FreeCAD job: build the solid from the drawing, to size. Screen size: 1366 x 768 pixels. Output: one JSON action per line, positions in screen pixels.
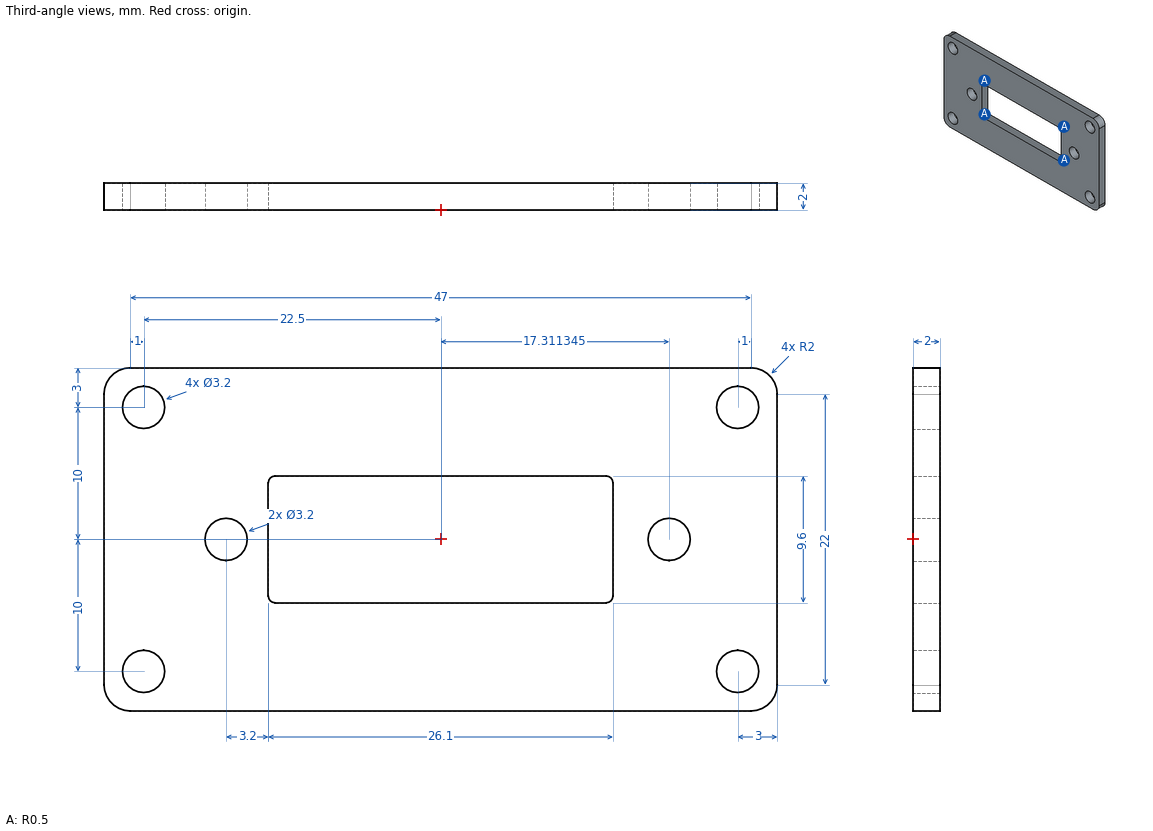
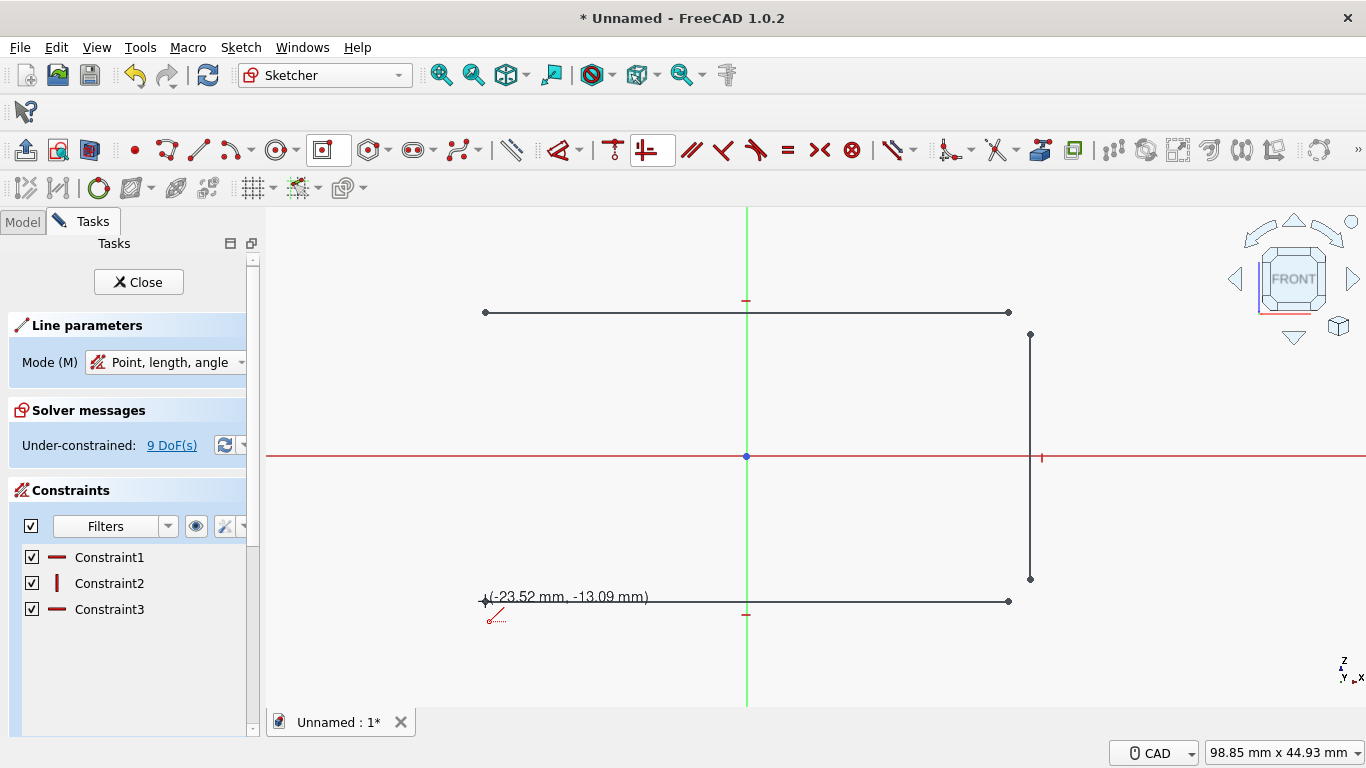
{"action": "left_click", "coordinate": [463, 579]}
{"action": "left_click", "coordinate": [463, 334]}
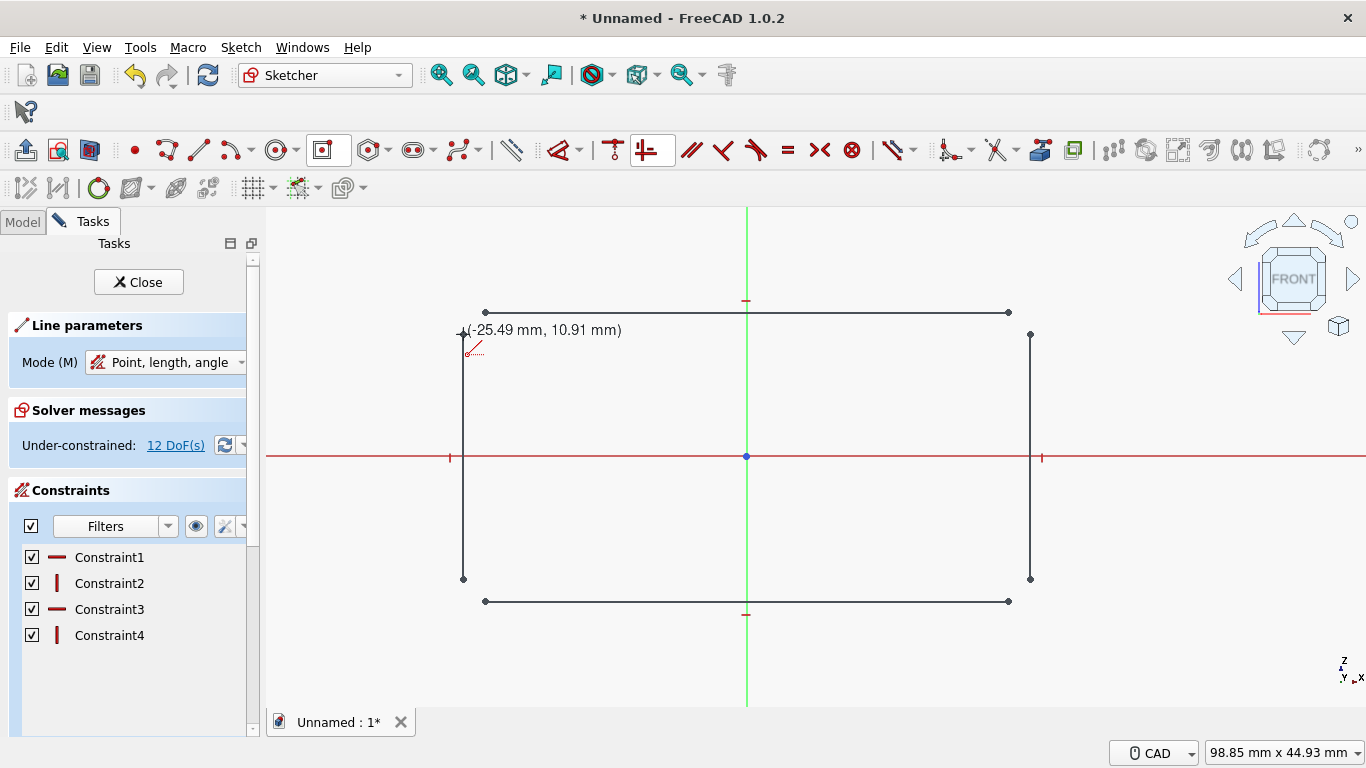
{"action": "key", "text": "g 3 a"}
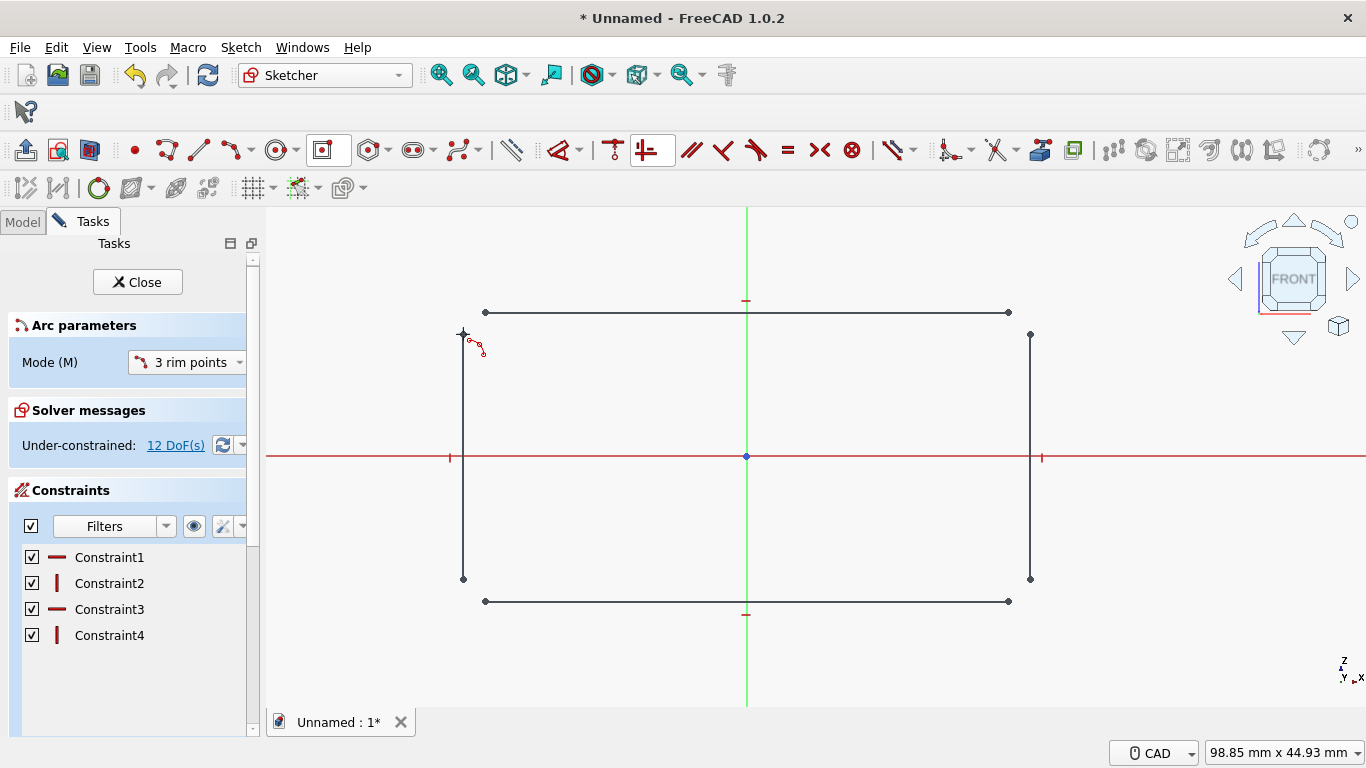
{"action": "left_click", "coordinate": [1008, 313]}
{"action": "left_click", "coordinate": [1030, 335]}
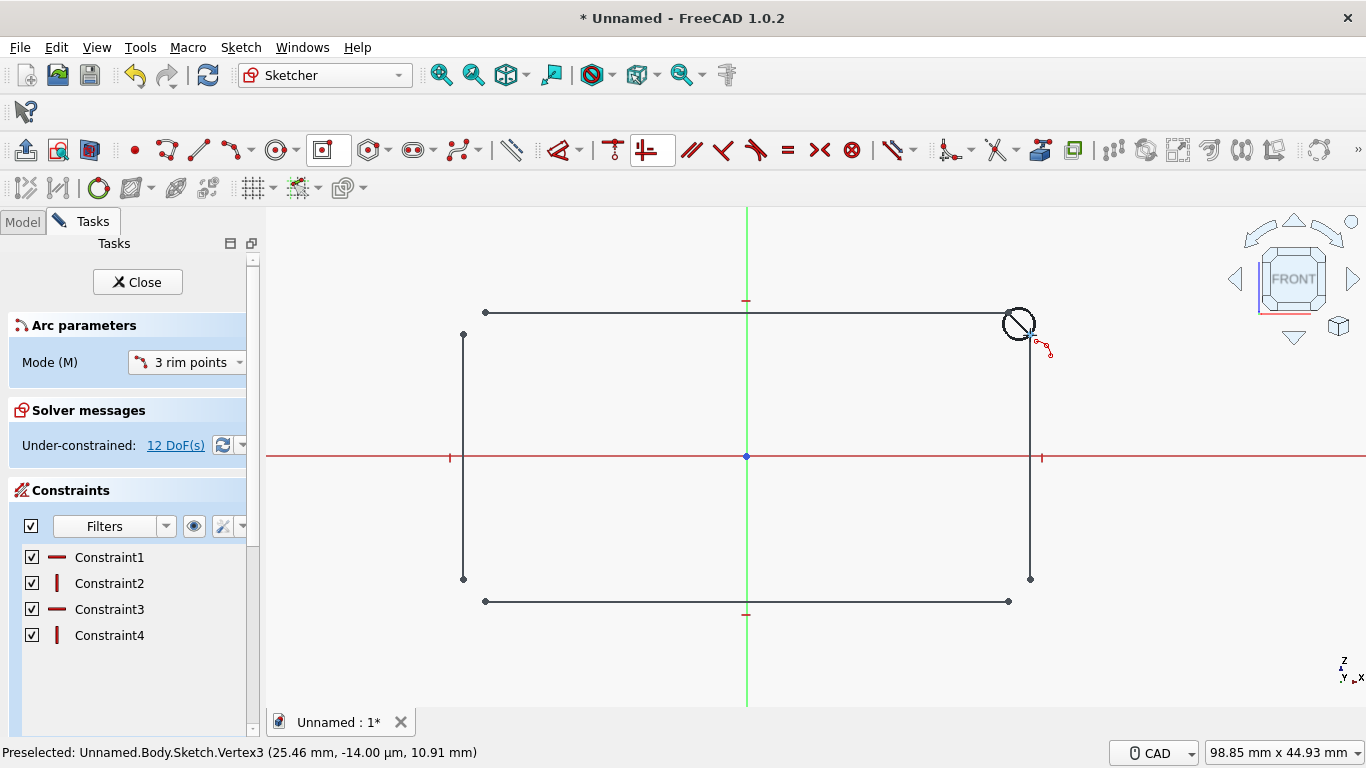
{"action": "scroll", "coordinate": [1024, 318], "scroll_direction": "up", "scroll_amount": 5}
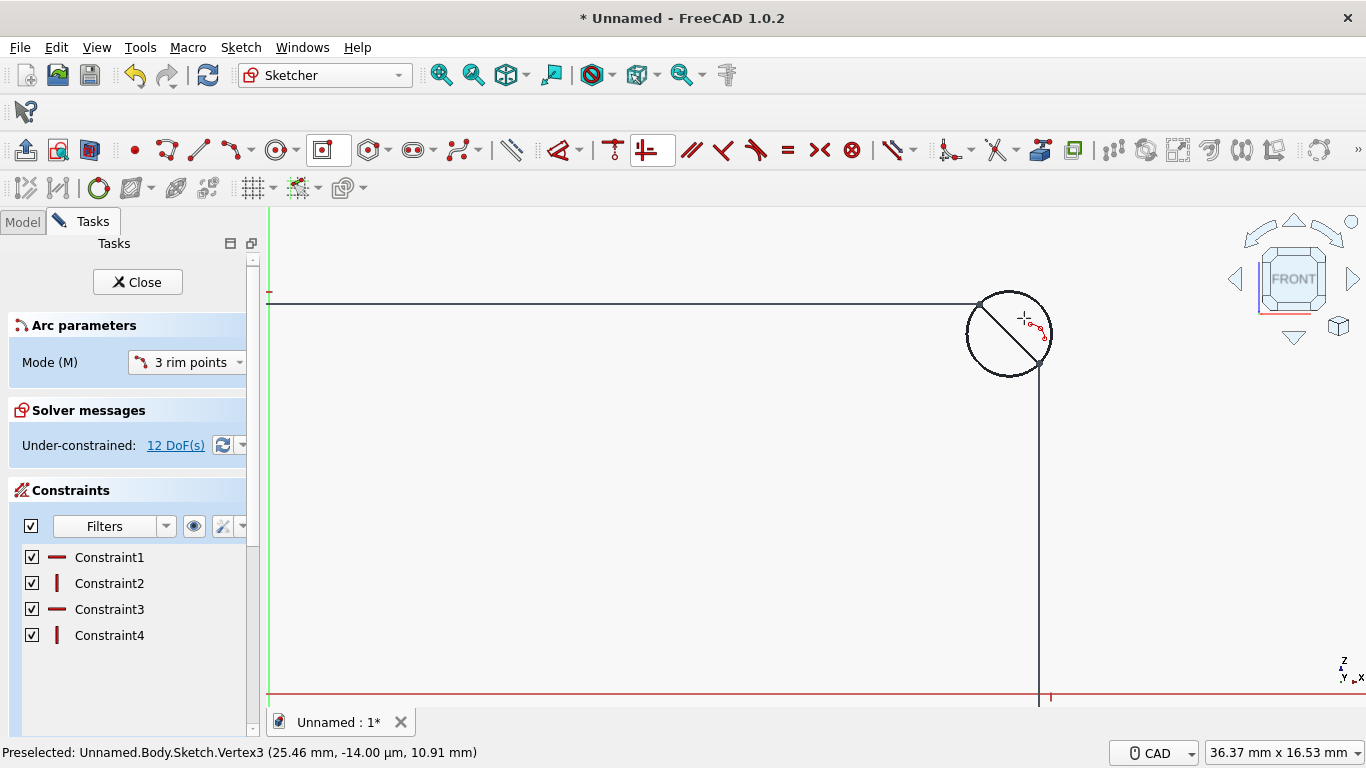
{"action": "left_click", "coordinate": [1023, 318]}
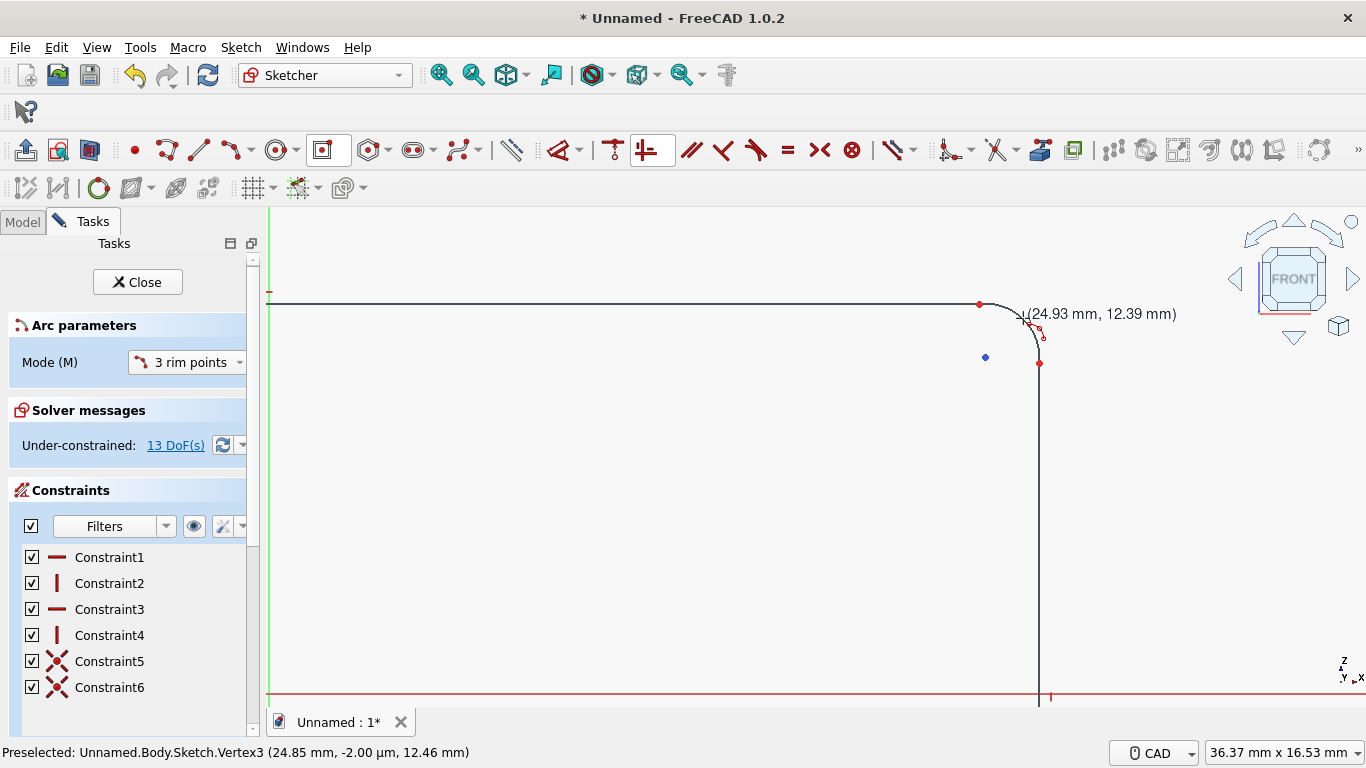
{"action": "scroll", "coordinate": [1026, 319], "scroll_direction": "down", "scroll_amount": 5}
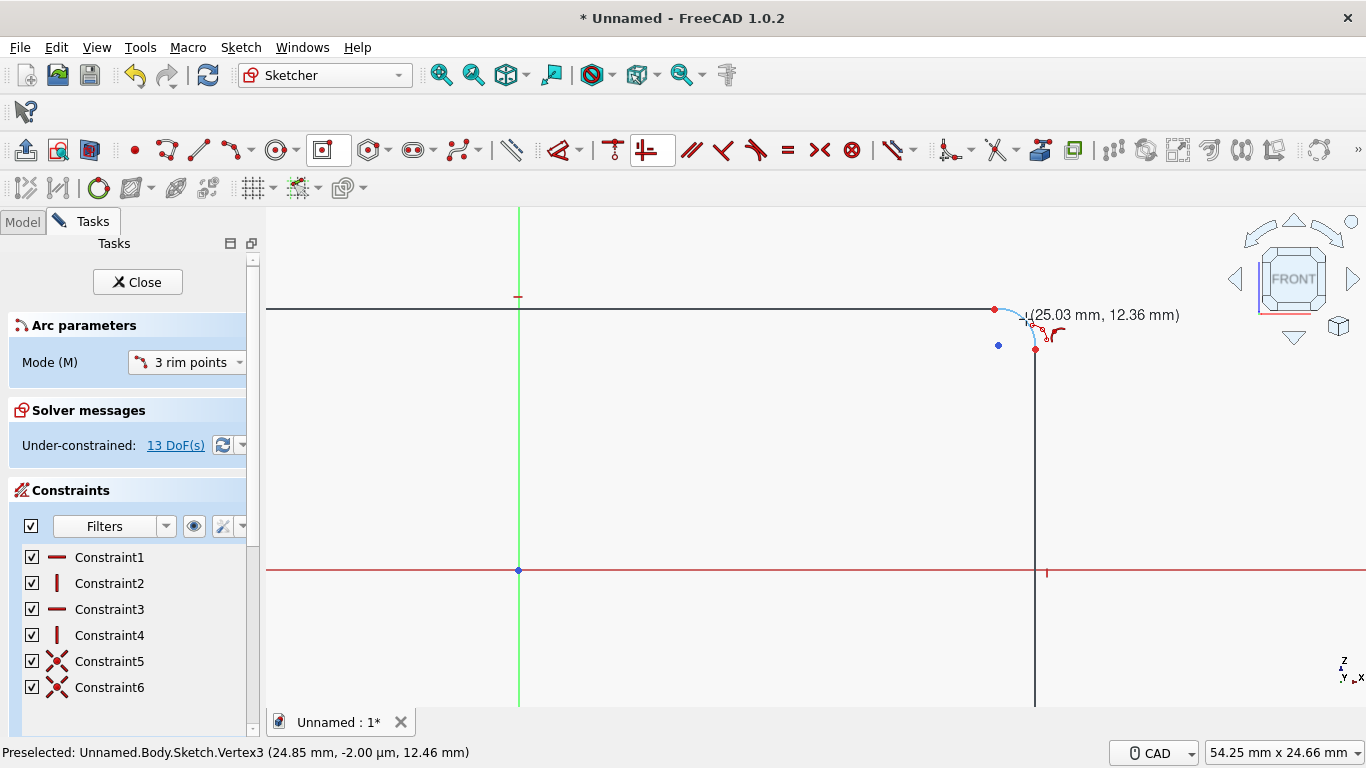
{"action": "left_click", "coordinate": [1031, 581]}
{"action": "left_click", "coordinate": [1009, 603]}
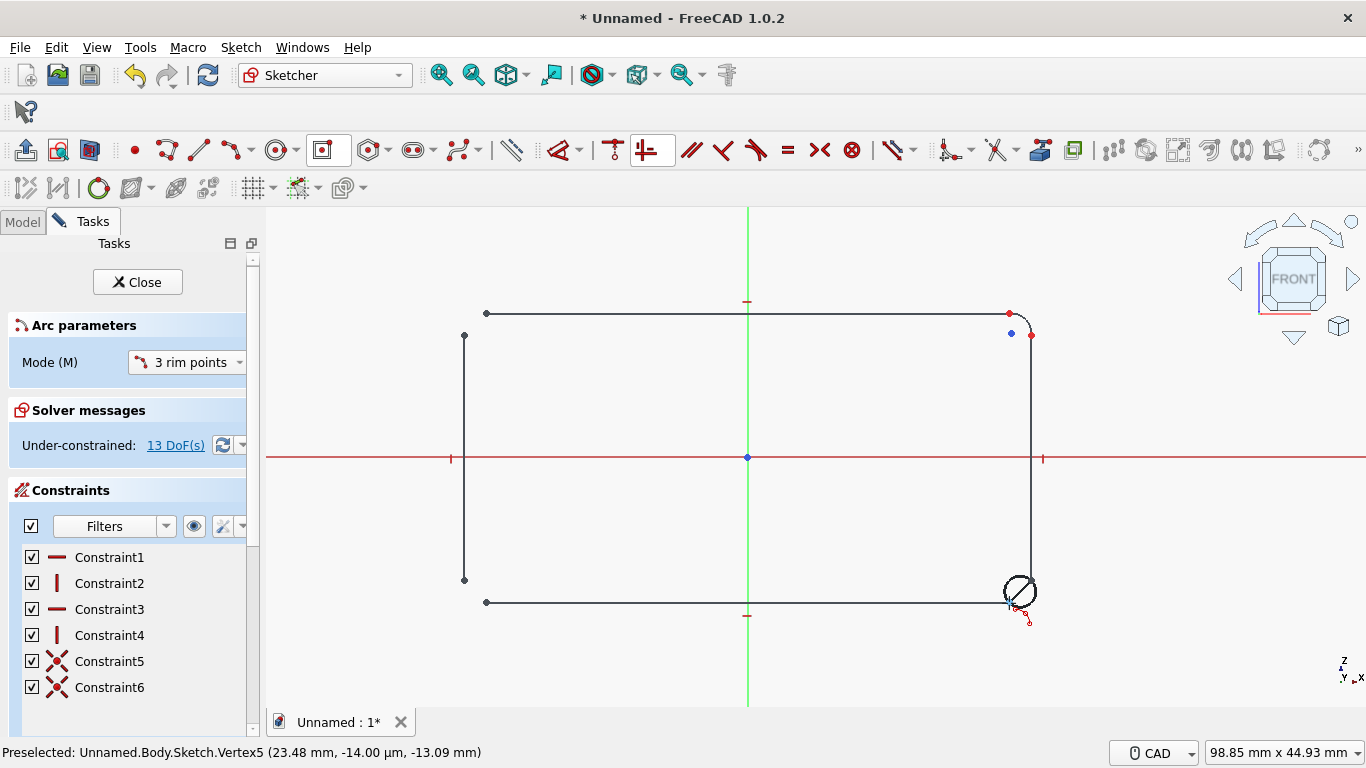
{"action": "scroll", "coordinate": [1025, 595], "scroll_direction": "up", "scroll_amount": 5}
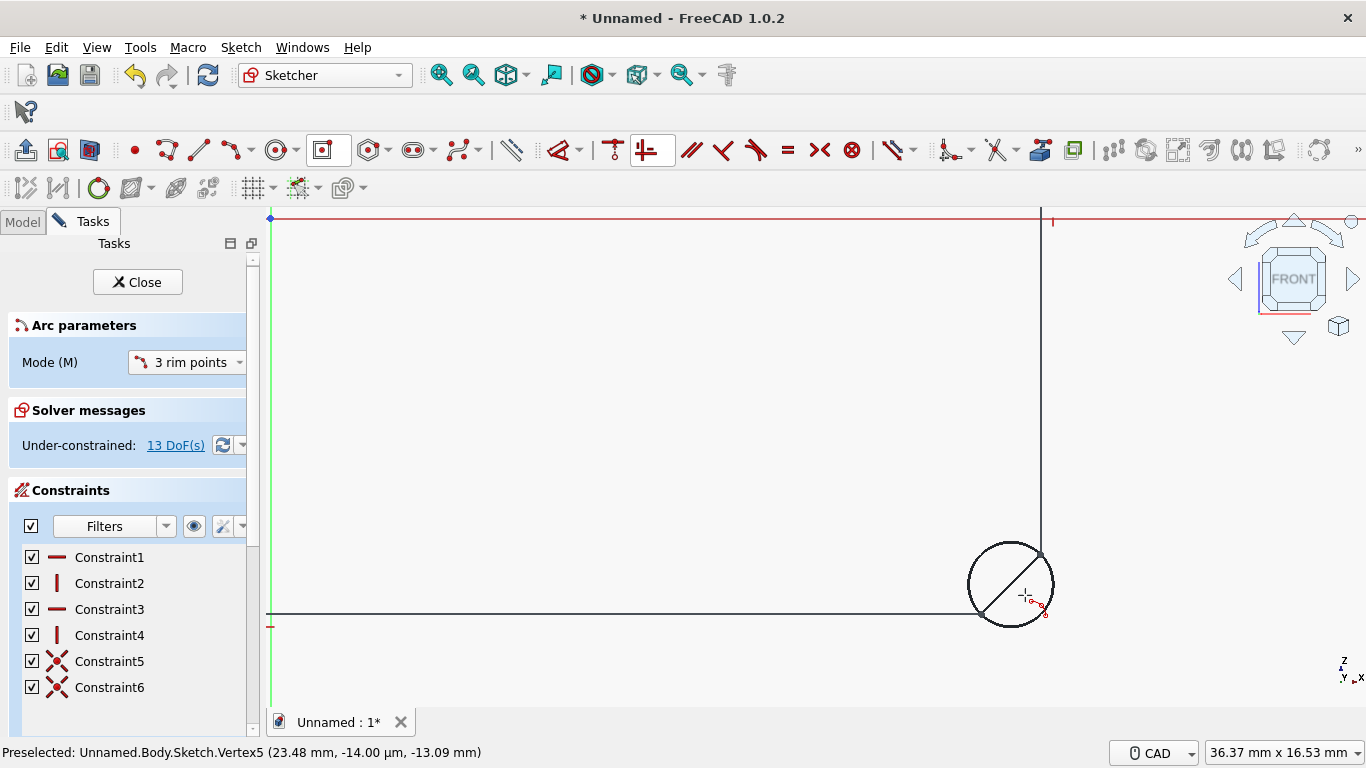
{"action": "left_click", "coordinate": [1024, 594]}